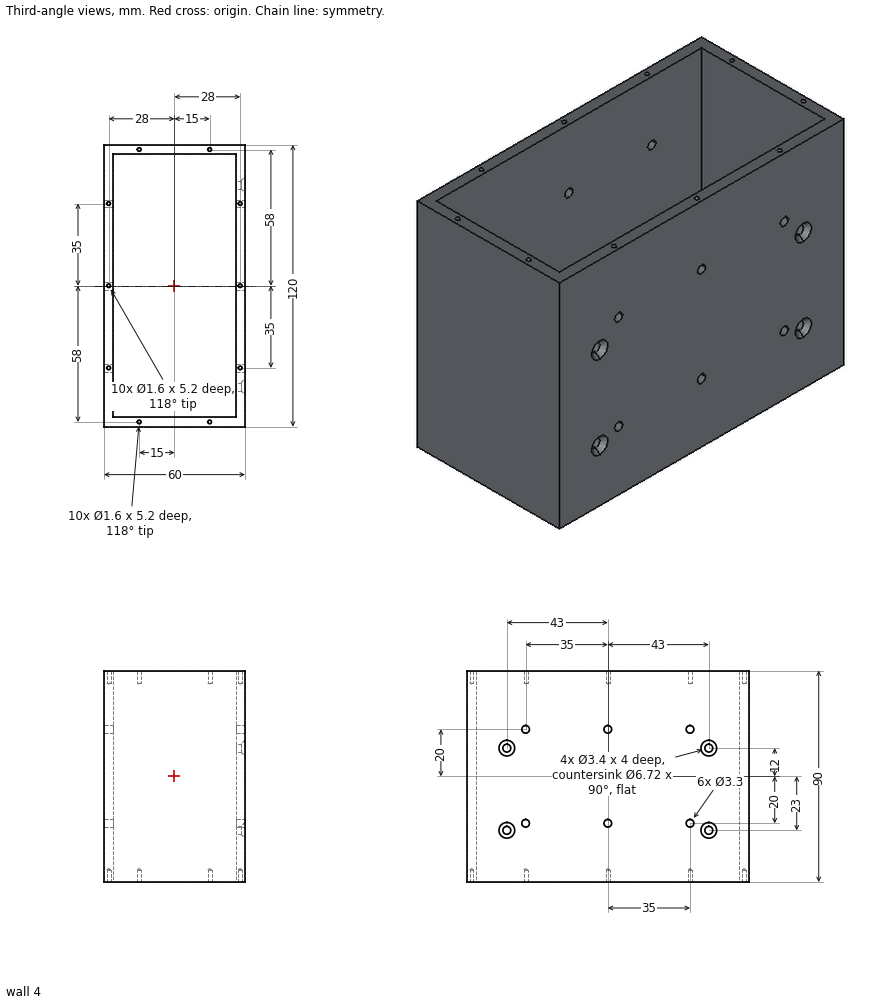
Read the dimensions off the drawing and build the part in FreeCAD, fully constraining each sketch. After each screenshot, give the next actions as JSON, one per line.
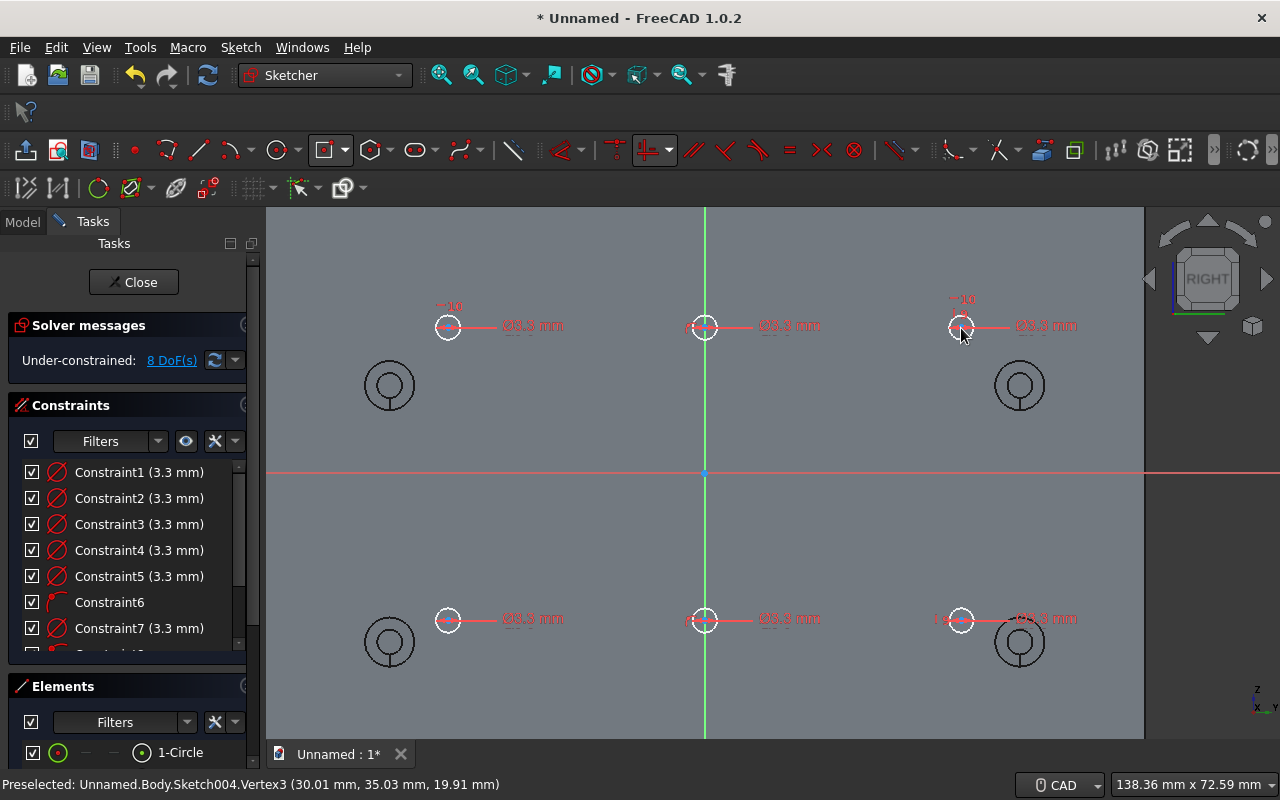
{"action": "left_click", "coordinate": [448, 328]}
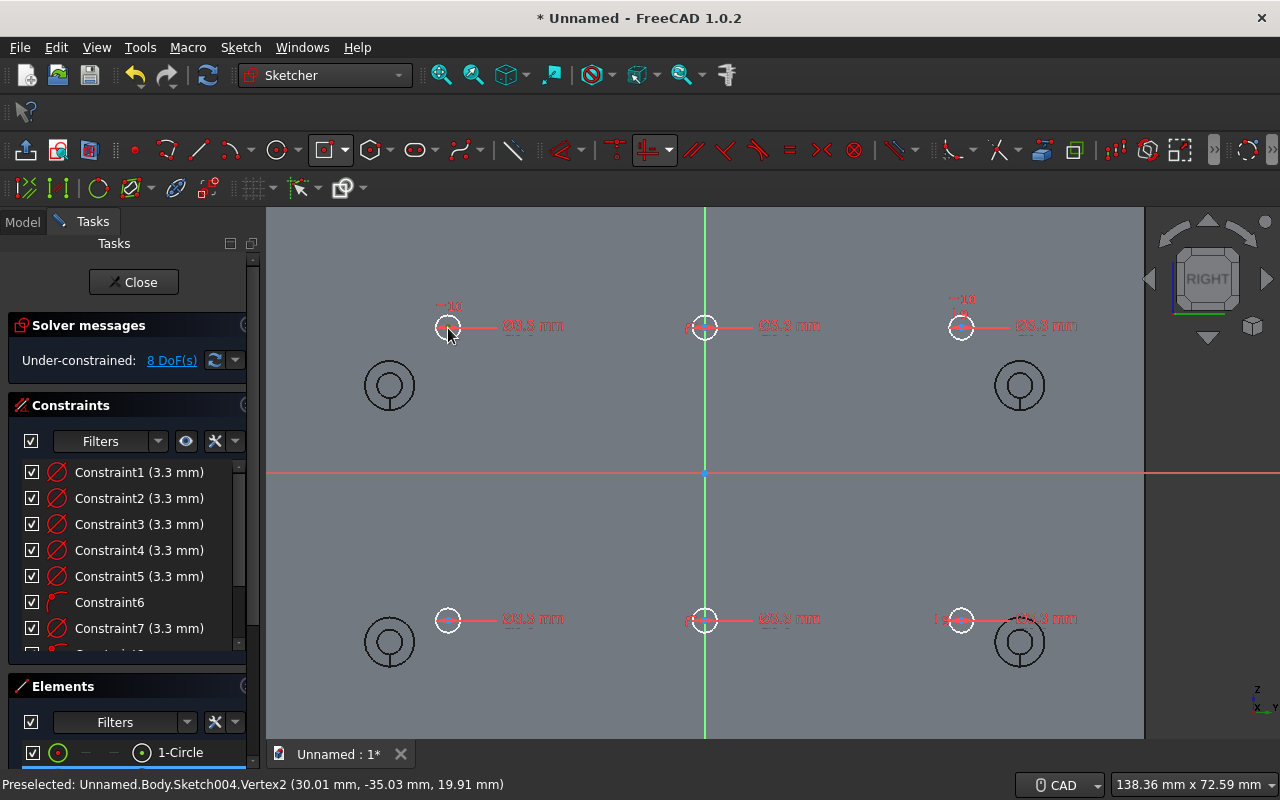
{"action": "left_click", "coordinate": [448, 621]}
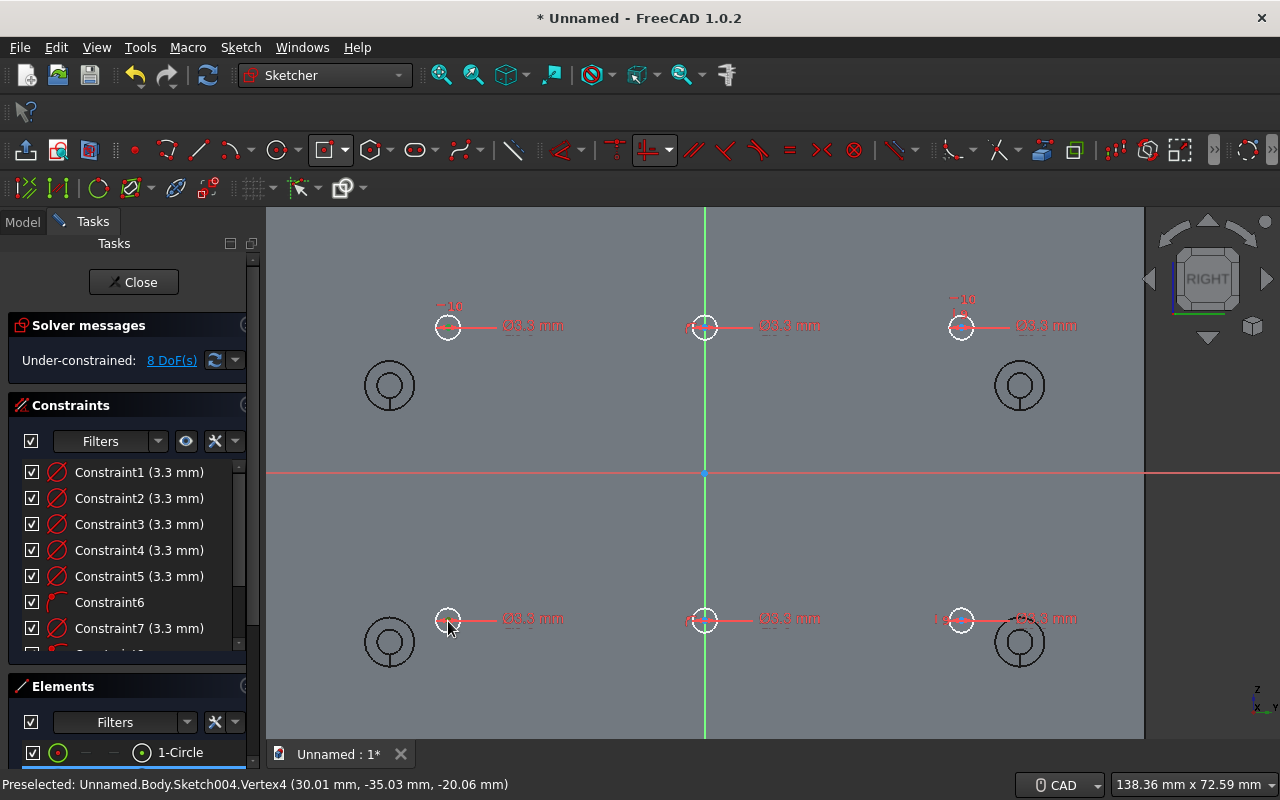
{"action": "left_click", "coordinate": [672, 150]}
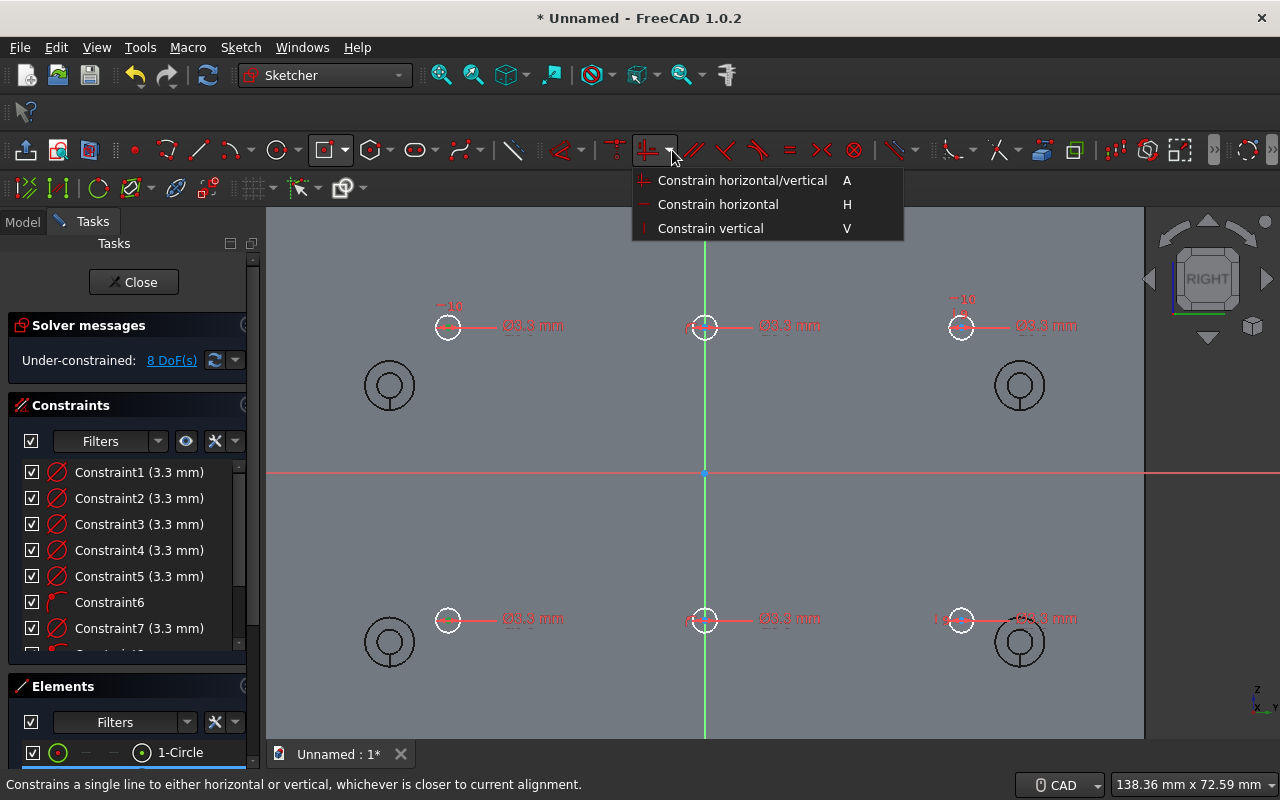
{"action": "left_click", "coordinate": [768, 228]}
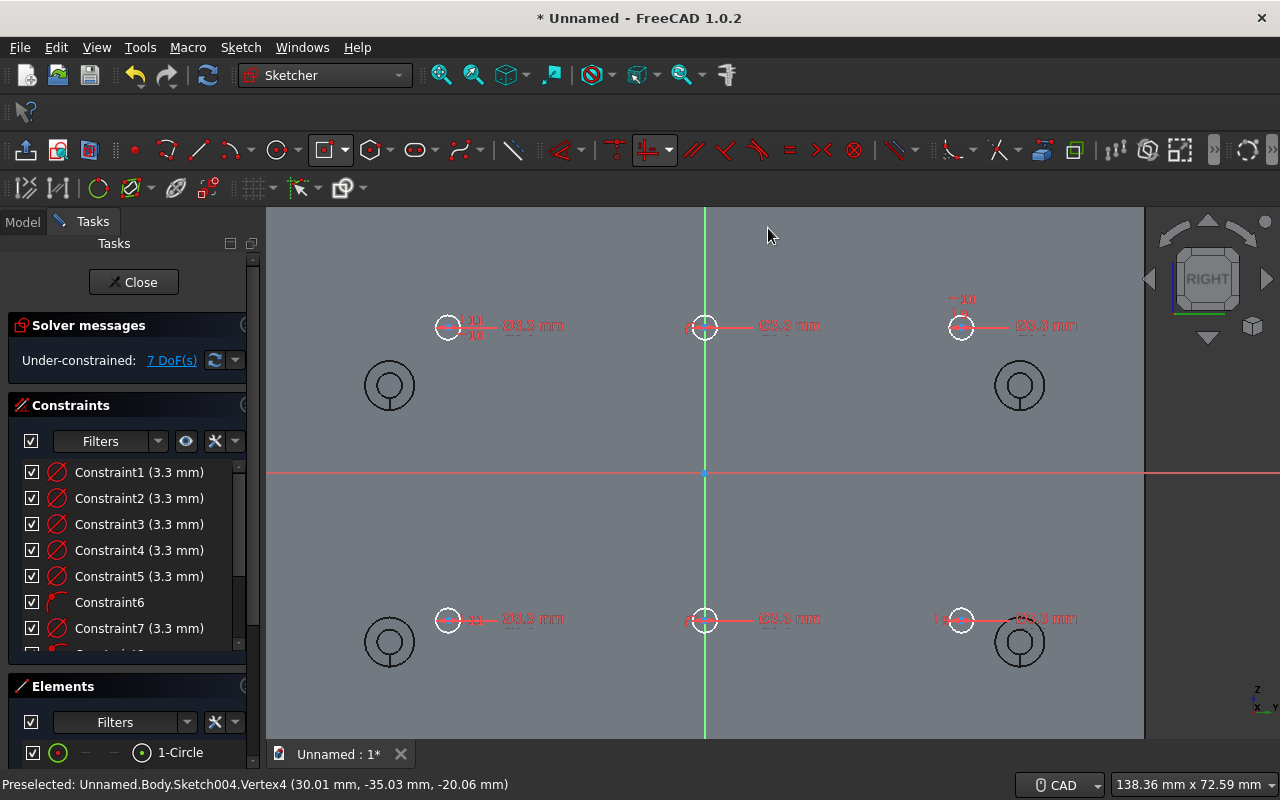
{"action": "left_click", "coordinate": [961, 621]}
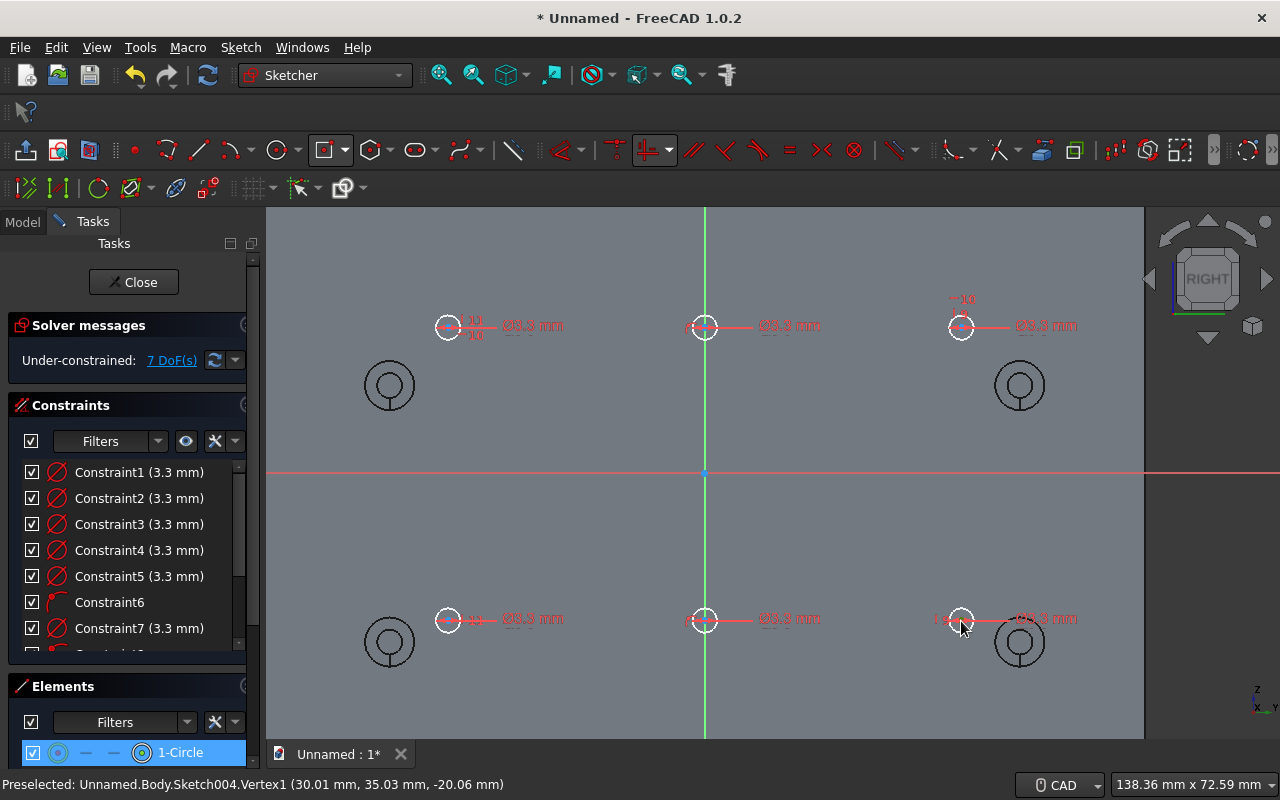
{"action": "left_click", "coordinate": [448, 621]}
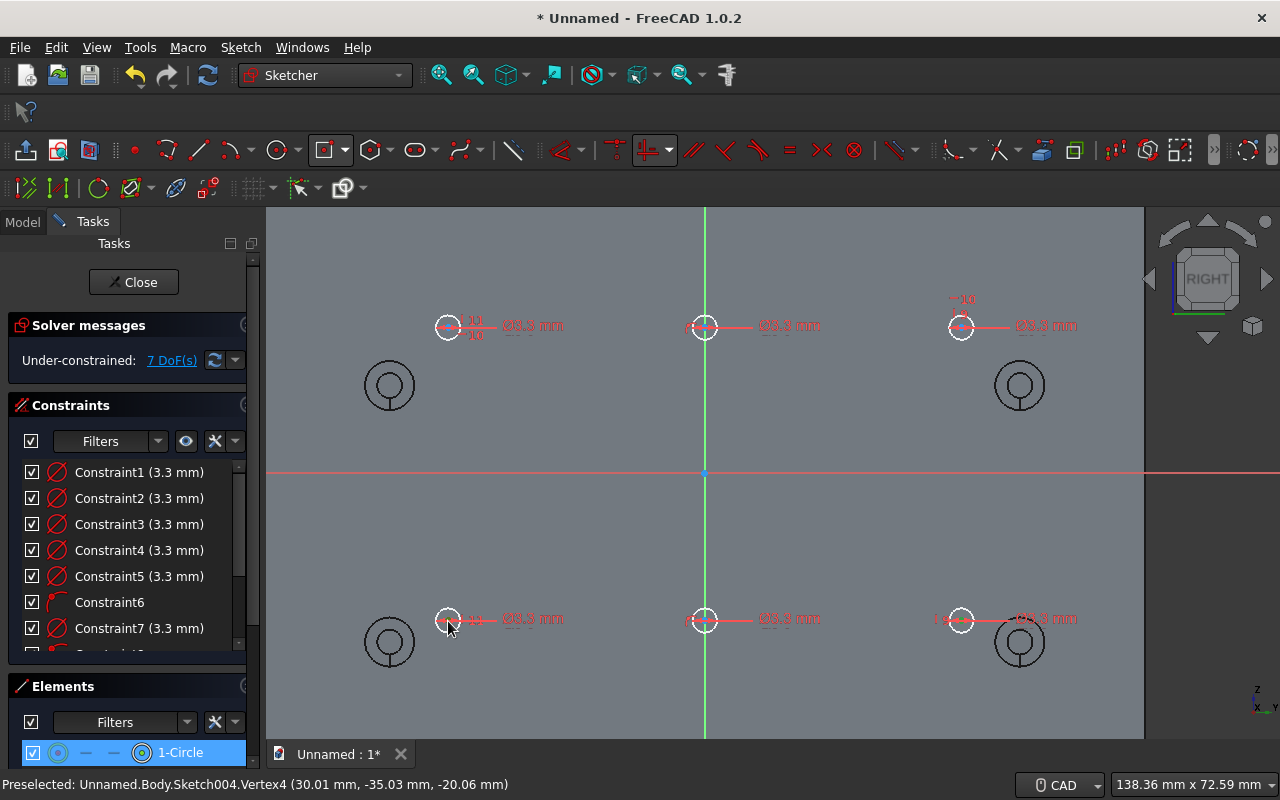
{"action": "key", "text": "h"}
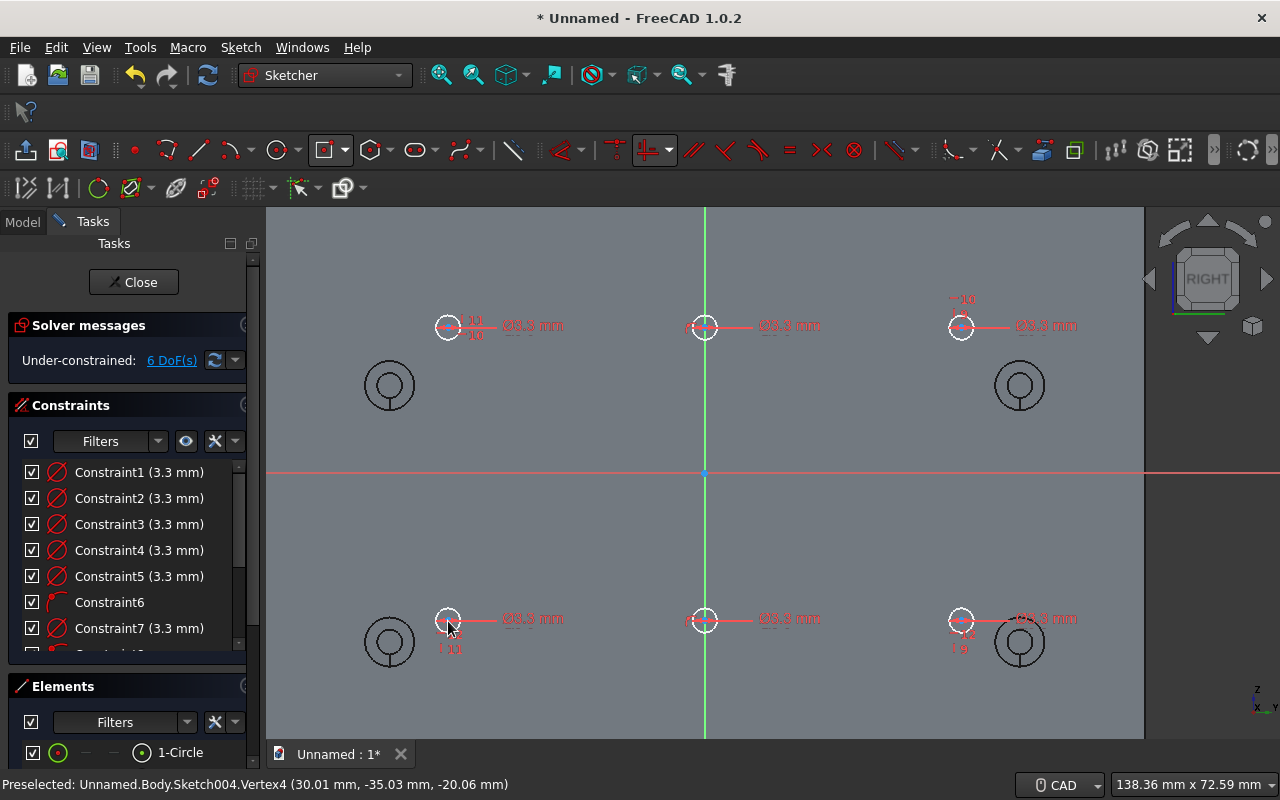
{"action": "left_click", "coordinate": [448, 328]}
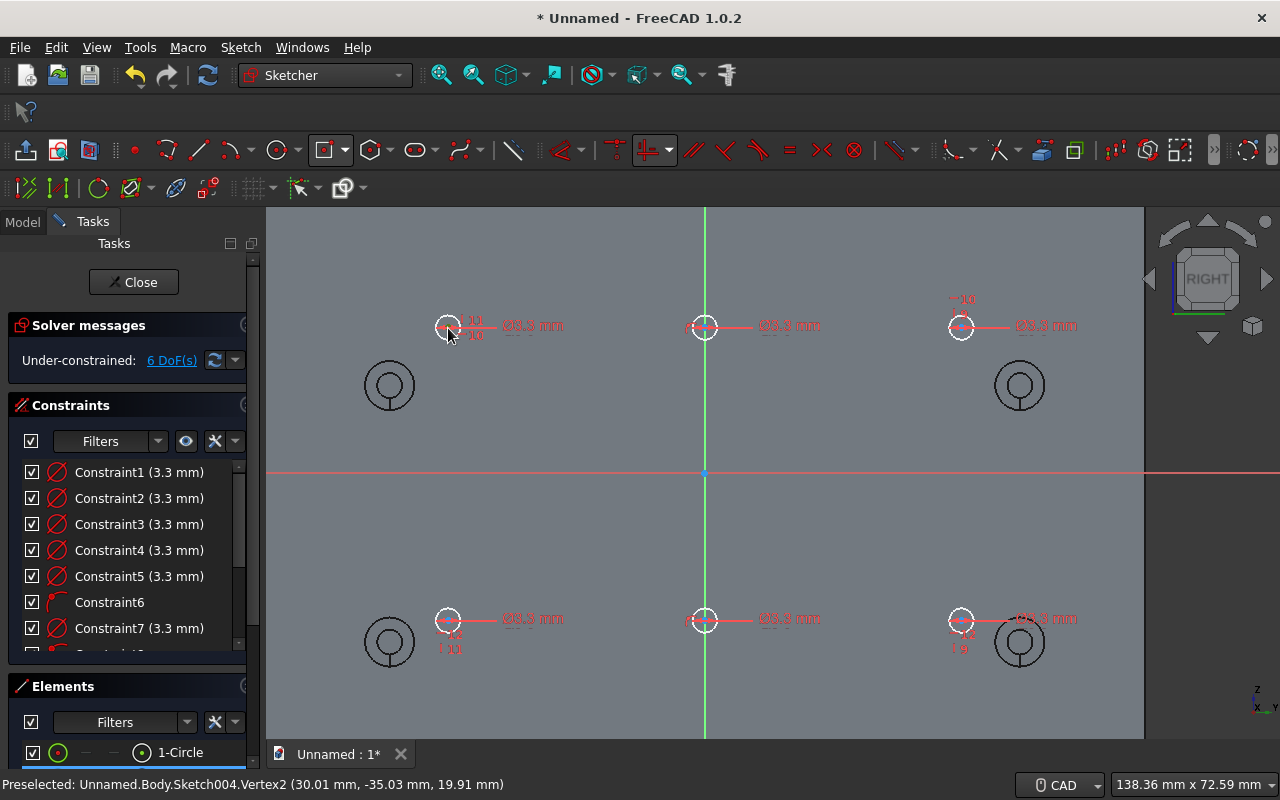
{"action": "left_click", "coordinate": [705, 328]}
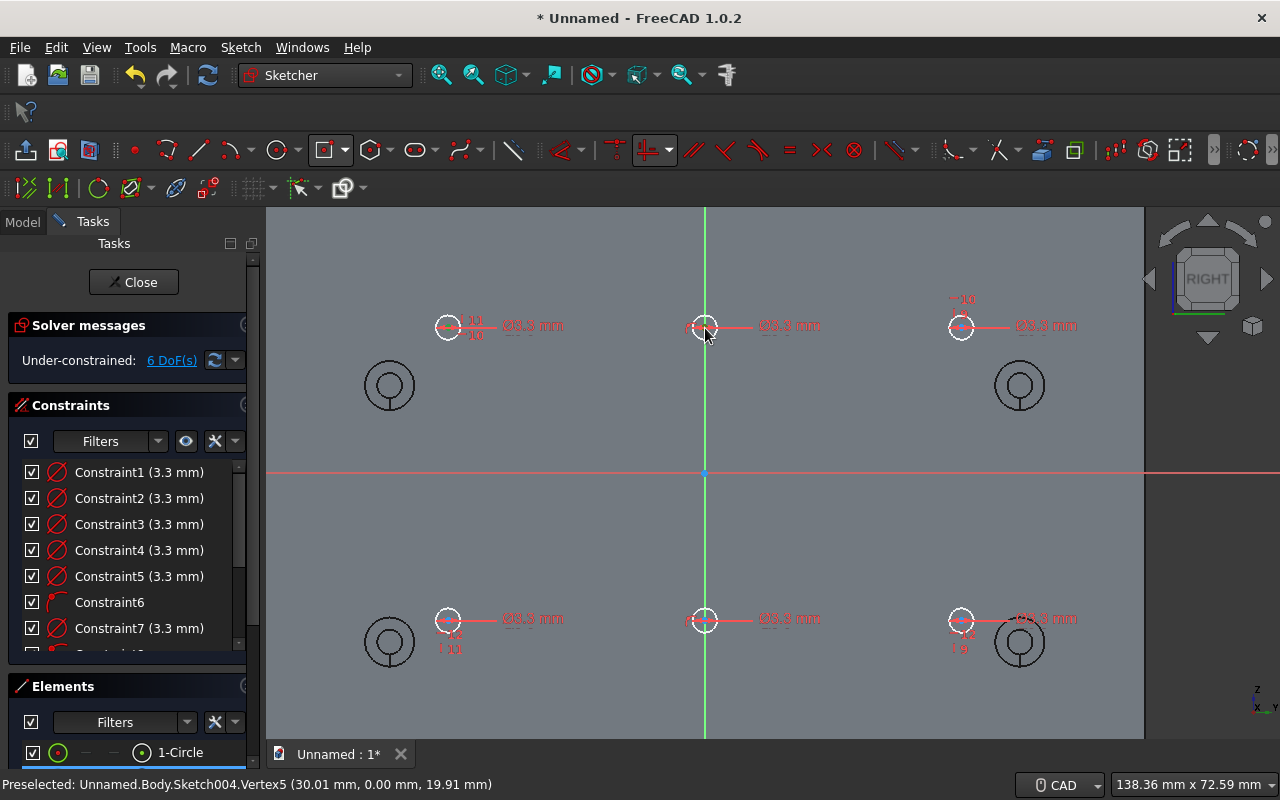
{"action": "left_click", "coordinate": [672, 150]}